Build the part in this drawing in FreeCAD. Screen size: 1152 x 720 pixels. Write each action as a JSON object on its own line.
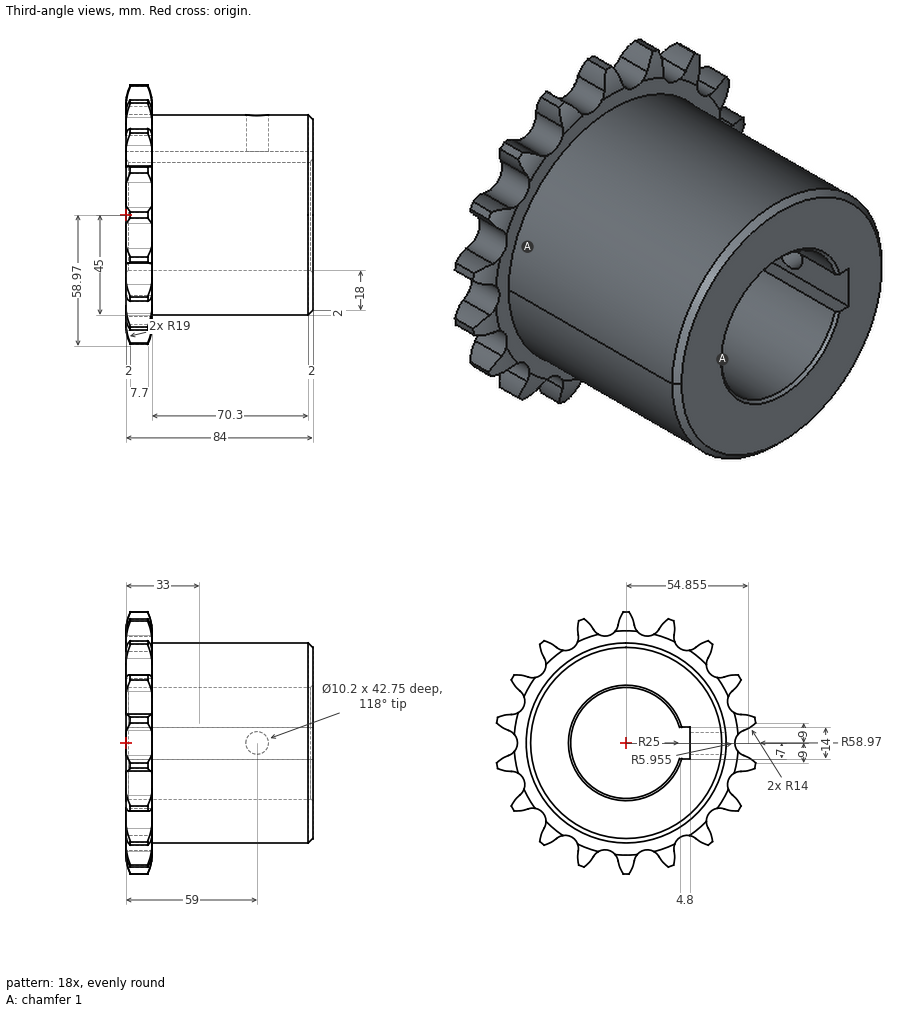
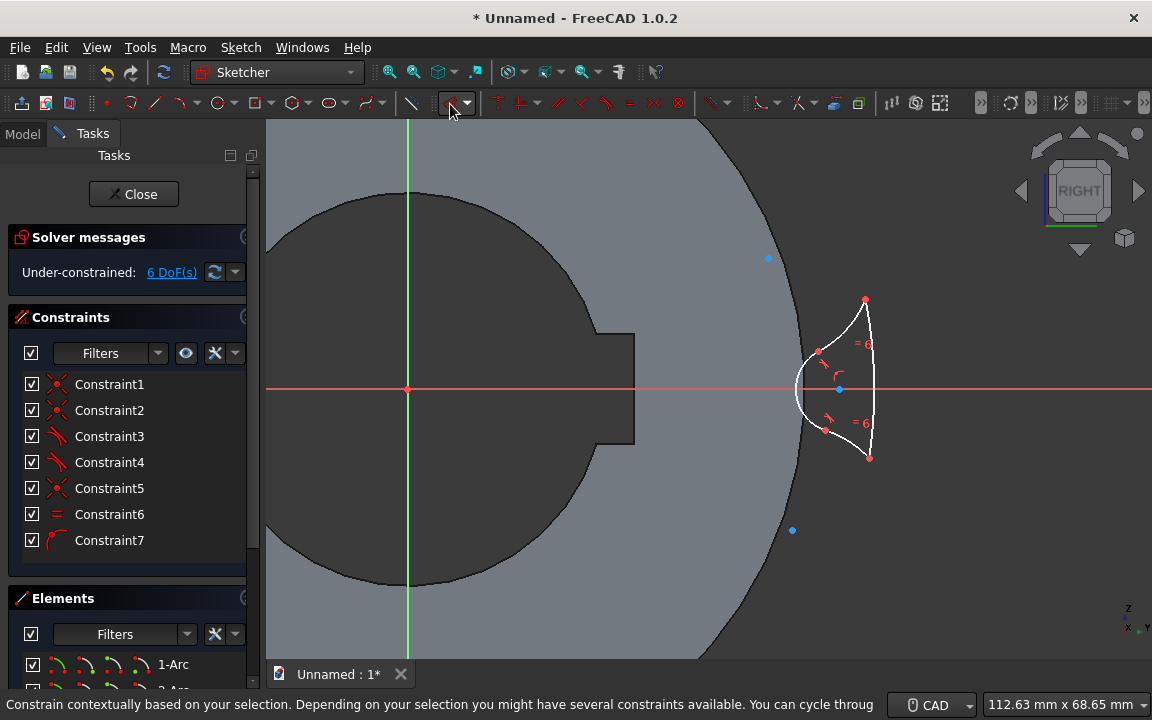
{"action": "left_click", "coordinate": [799, 374]}
{"action": "left_click", "coordinate": [769, 362]}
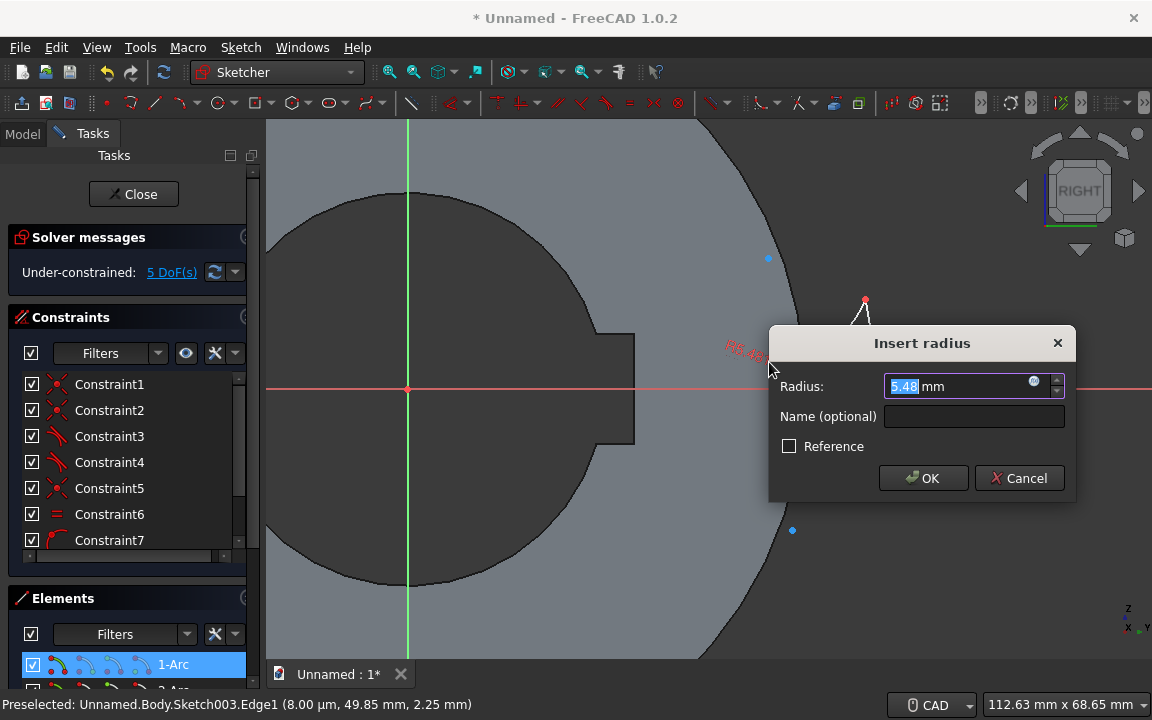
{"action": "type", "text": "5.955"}
{"action": "key", "text": "Return"}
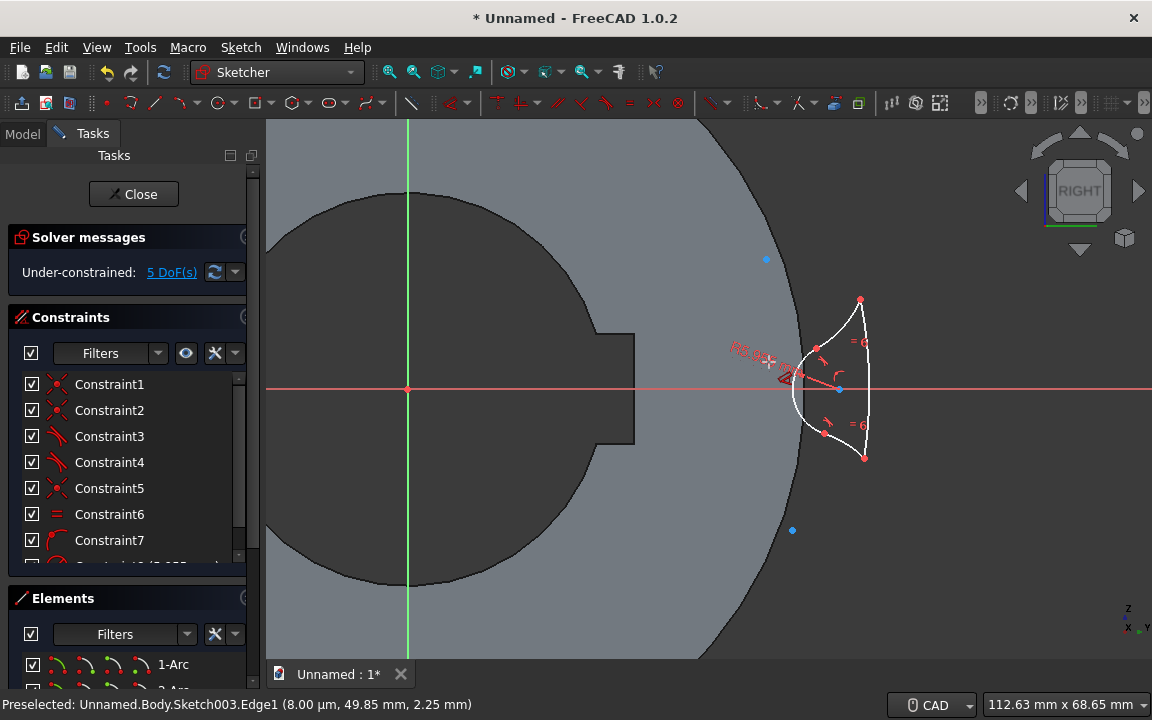
{"action": "left_click", "coordinate": [833, 337]}
{"action": "left_click", "coordinate": [854, 361]}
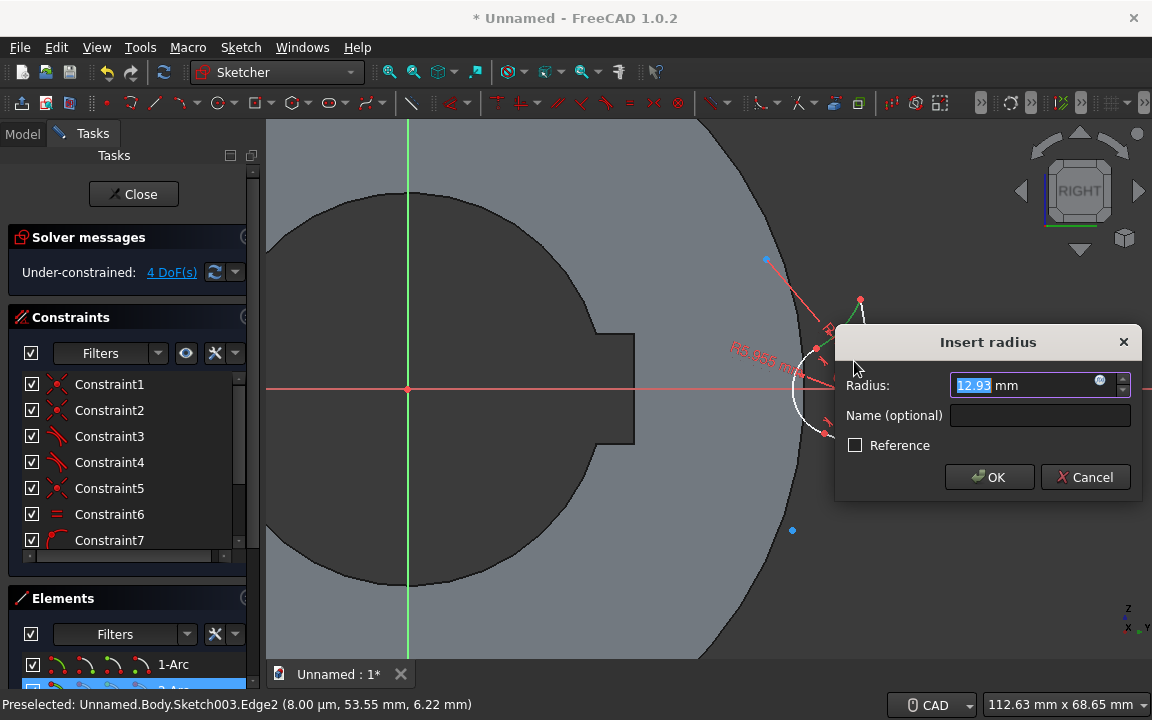
{"action": "type", "text": "14"}
{"action": "key", "text": "Return"}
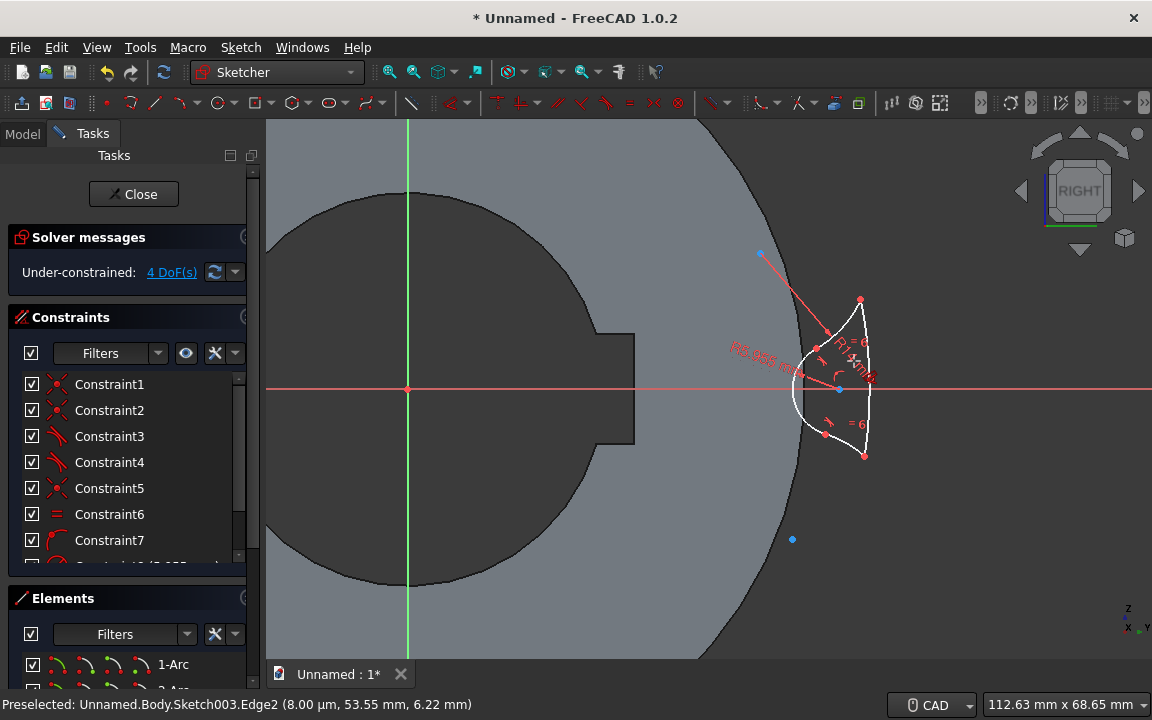
{"action": "left_click", "coordinate": [869, 409]}
{"action": "left_click", "coordinate": [901, 410]}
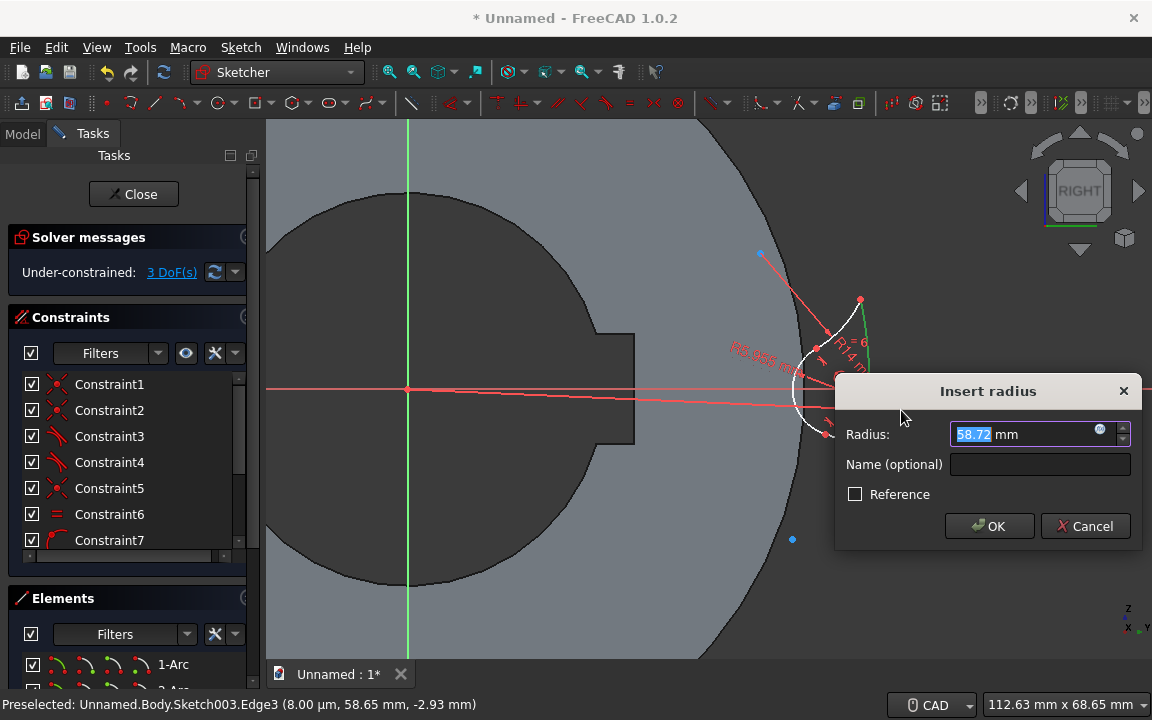
{"action": "type", "text": "58.97"}
{"action": "key", "text": "Return"}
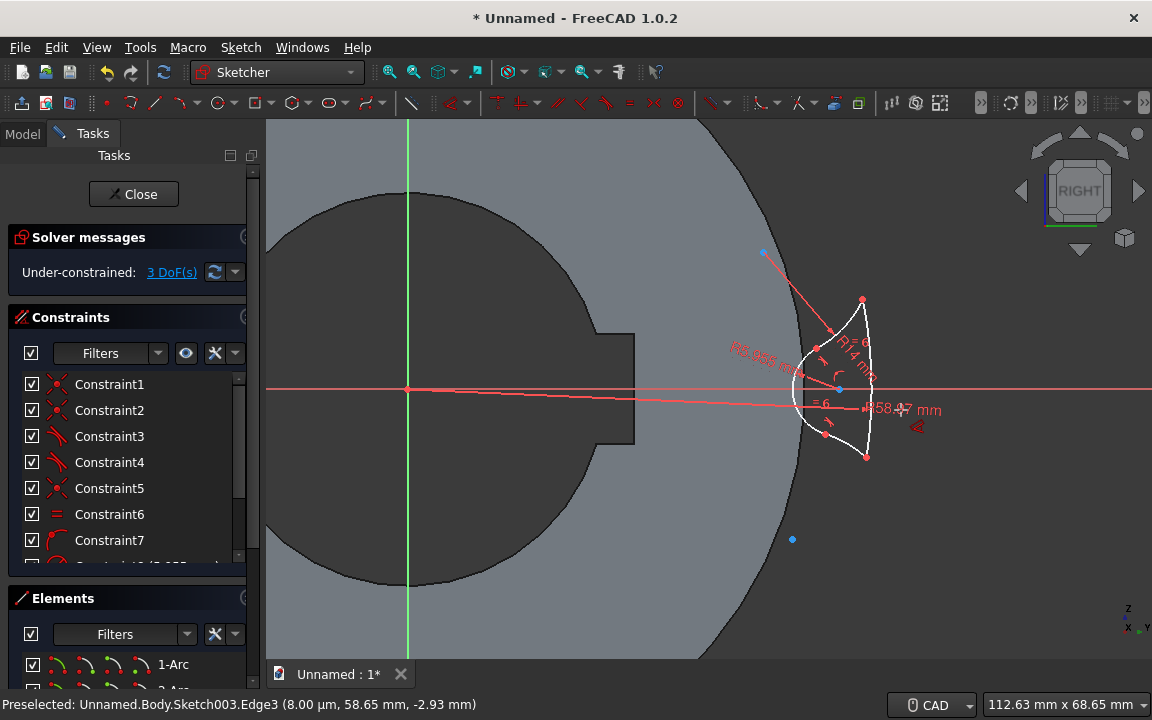
{"action": "left_click", "coordinate": [863, 300]}
{"action": "left_click", "coordinate": [374, 345]}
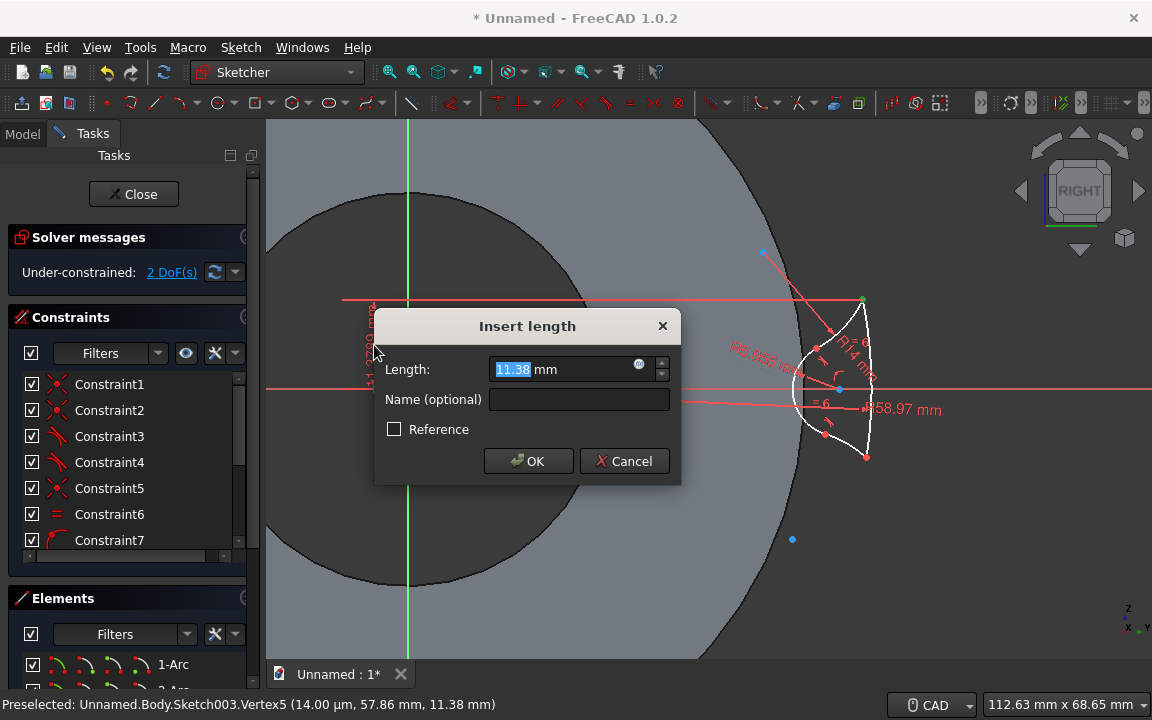
{"action": "type", "text": "9"}
{"action": "key", "text": "Return"}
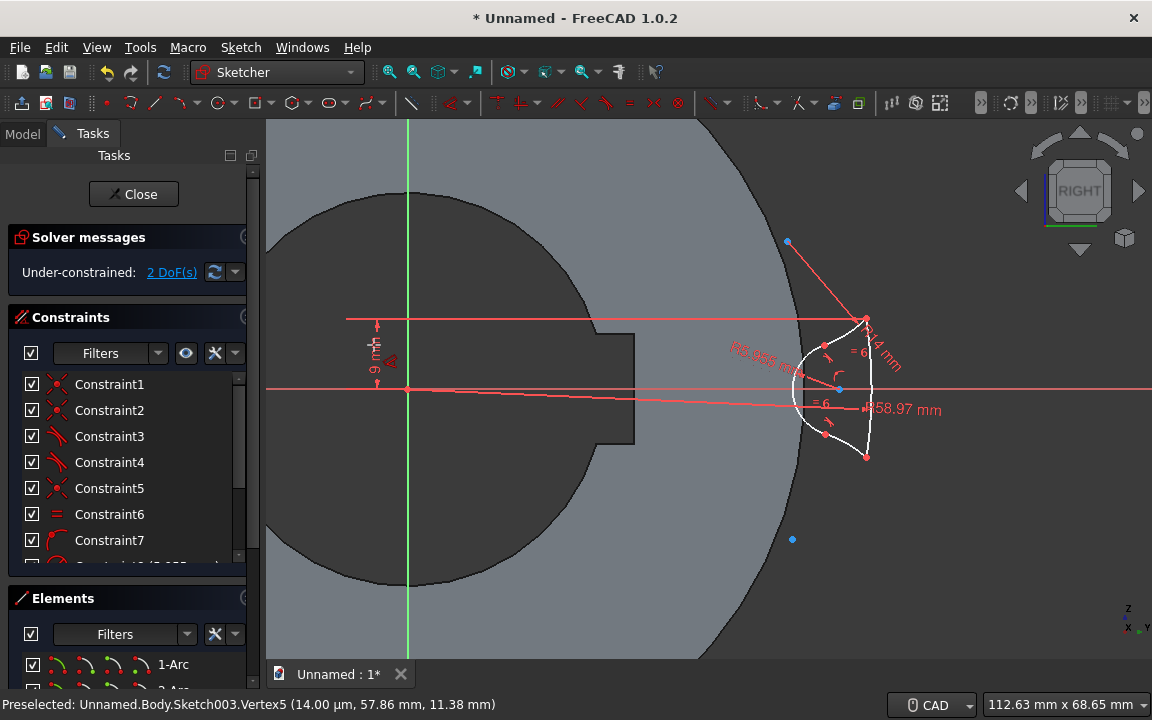
{"action": "left_click", "coordinate": [866, 458]}
{"action": "left_click", "coordinate": [374, 424]}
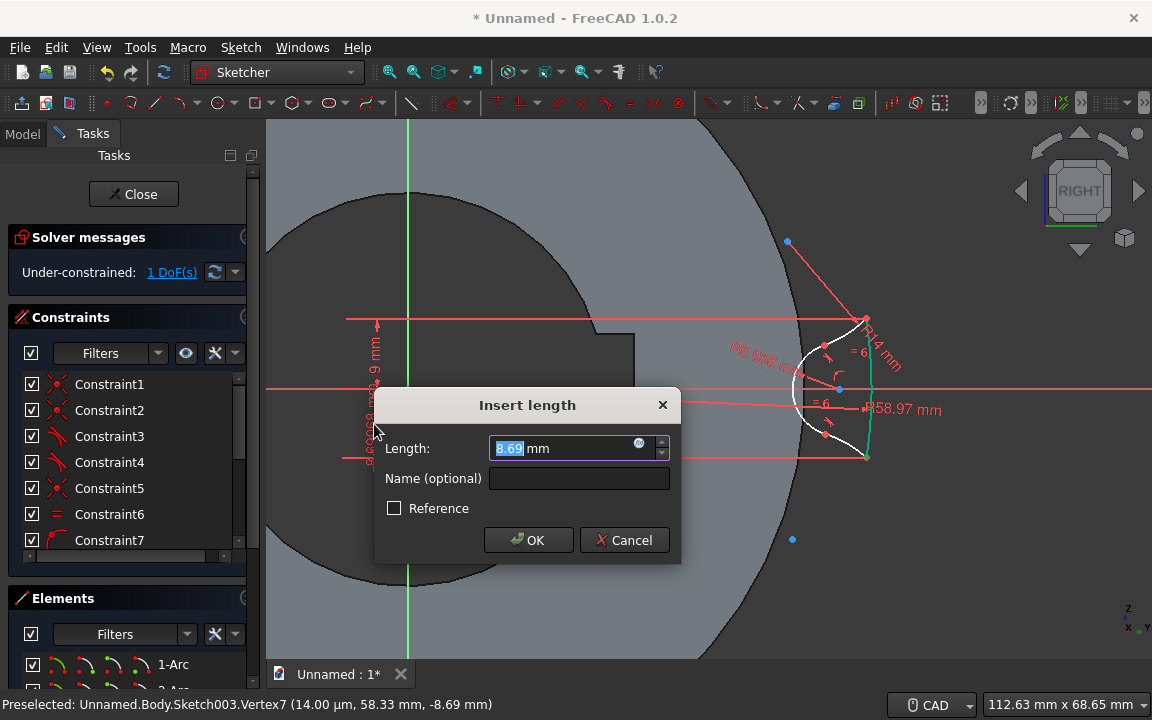
{"action": "type", "text": "9"}
{"action": "key", "text": "Return"}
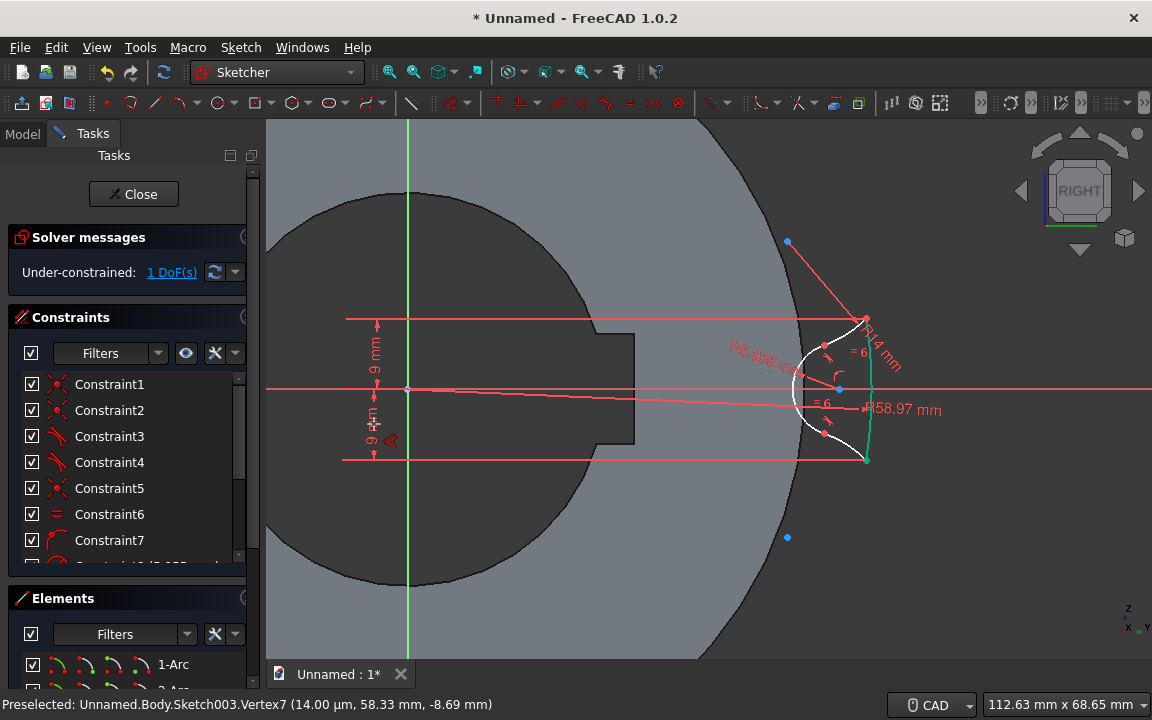
{"action": "left_click", "coordinate": [840, 389]}
{"action": "left_click", "coordinate": [624, 423]}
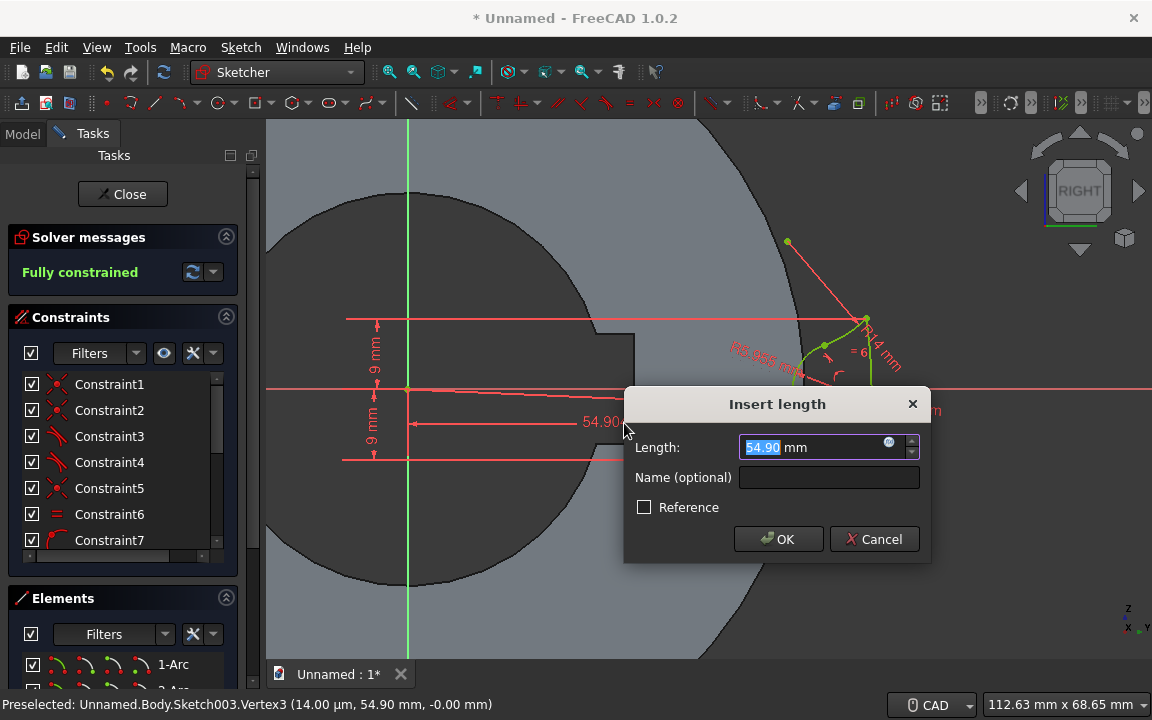
{"action": "type", "text": "54.855"}
{"action": "key", "text": "Return"}
{"action": "key", "text": "Escape"}